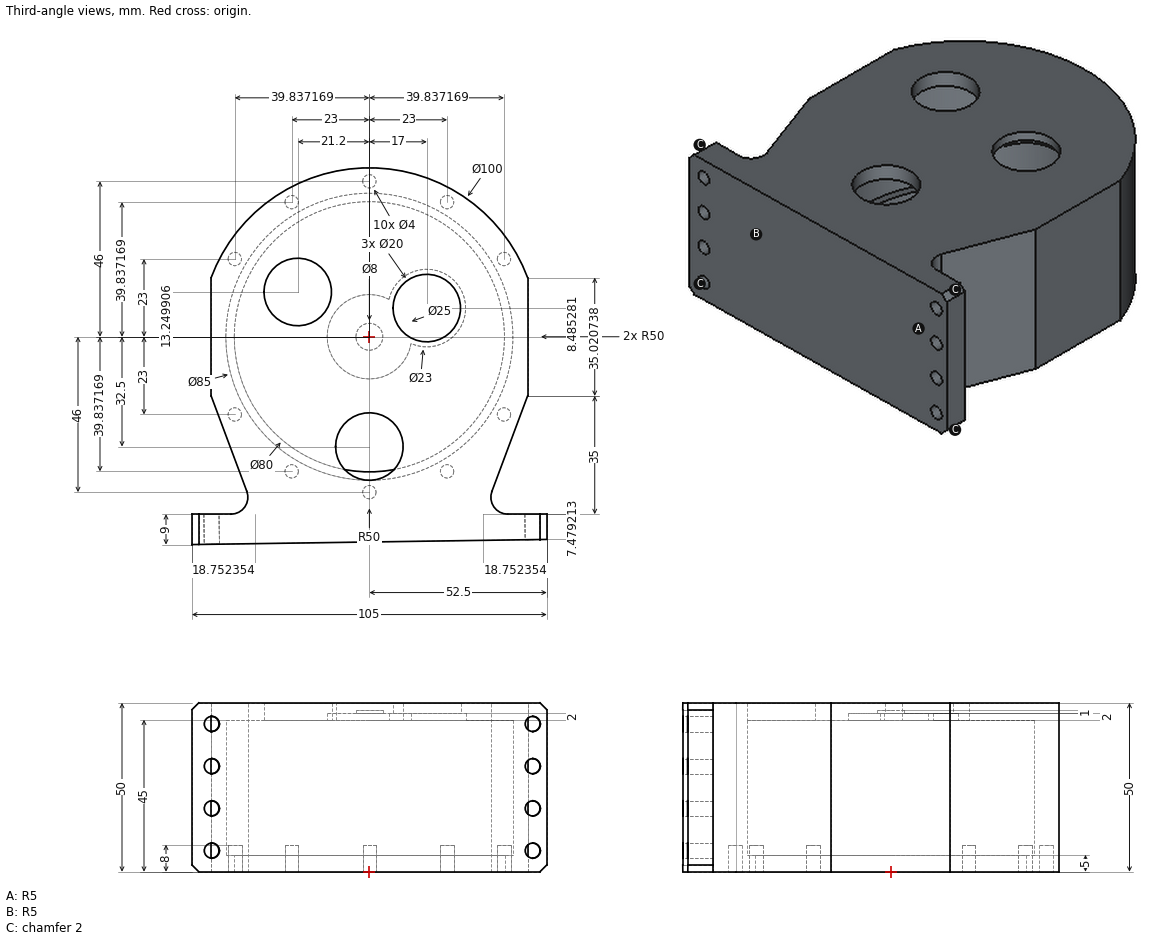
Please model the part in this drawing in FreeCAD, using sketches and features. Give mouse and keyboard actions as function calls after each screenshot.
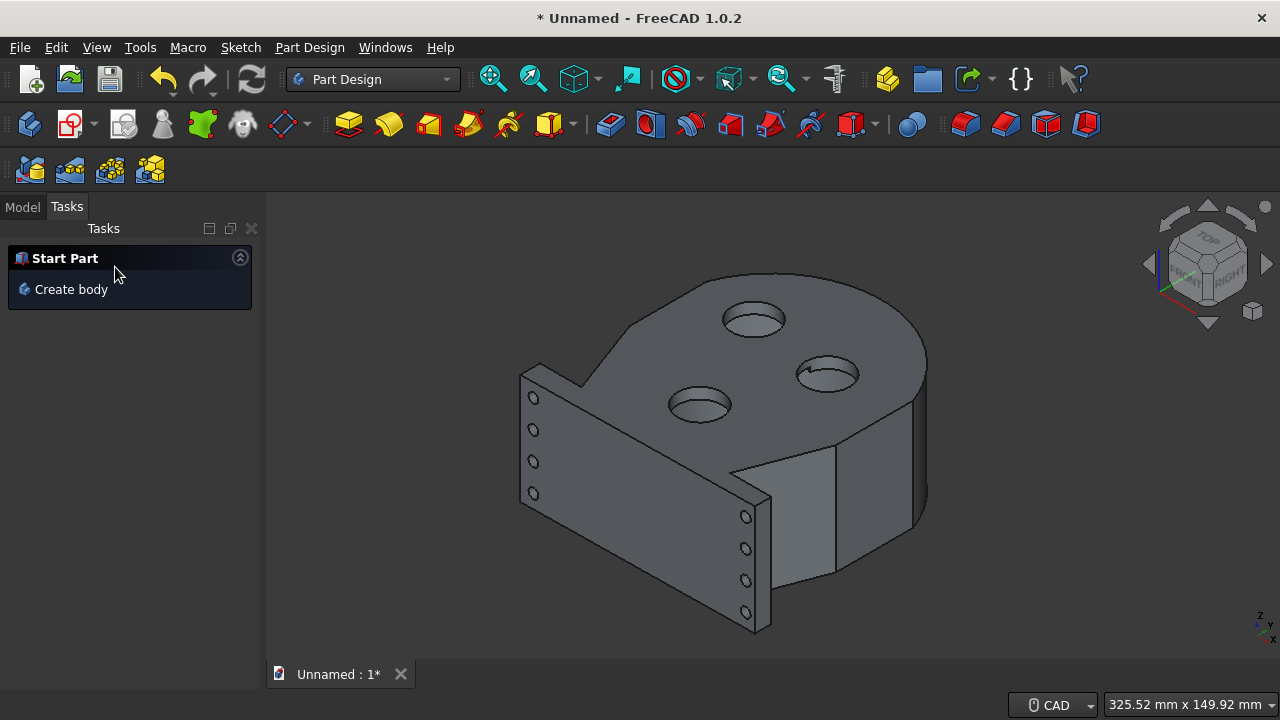
key(1)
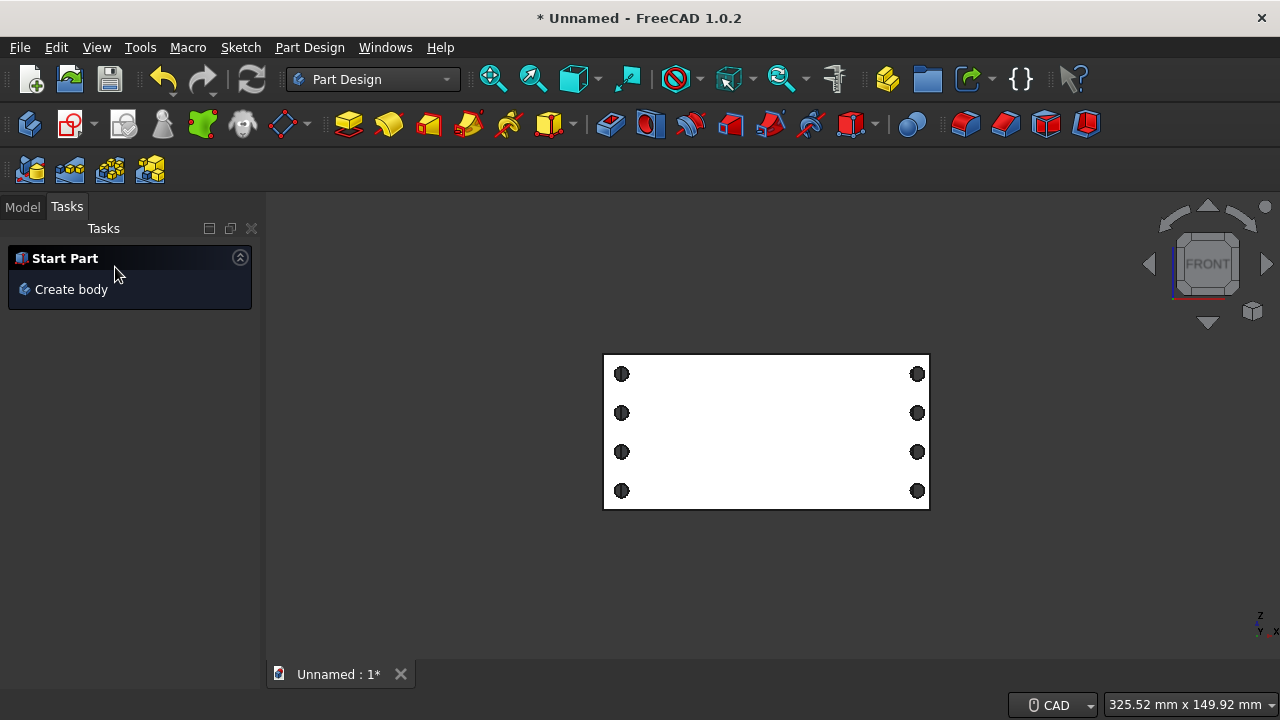
click(494, 80)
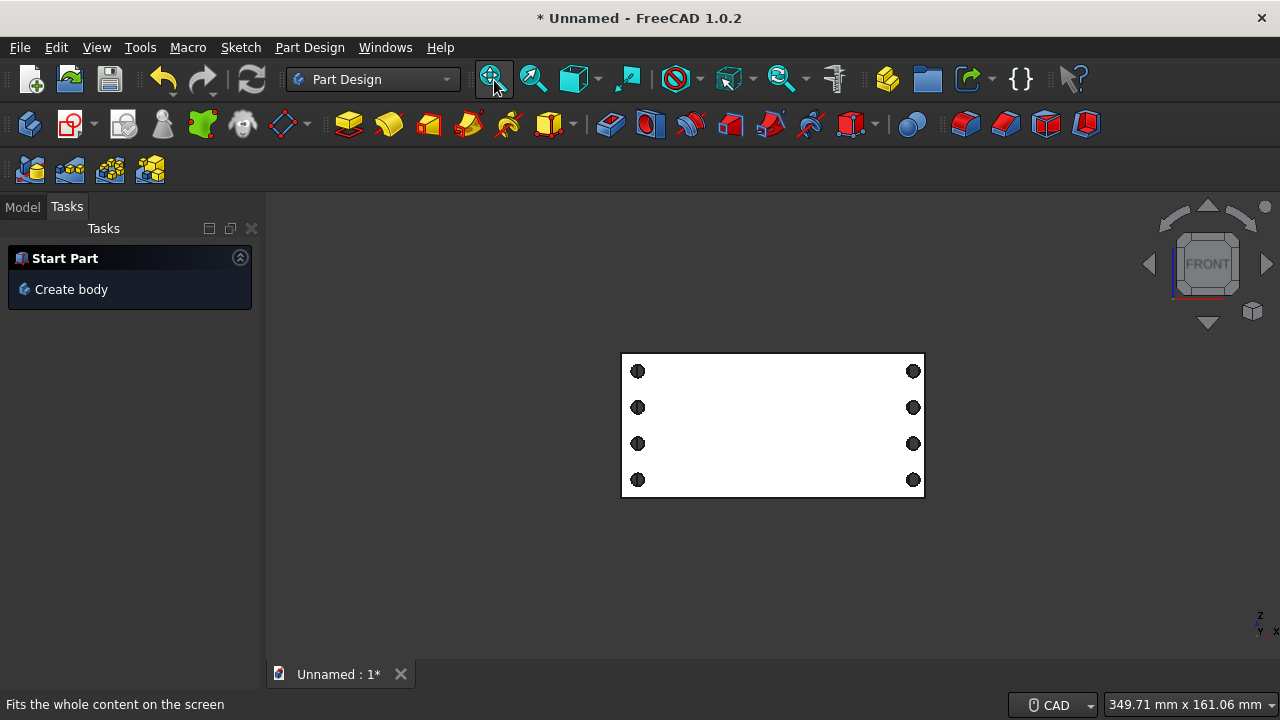
key(3)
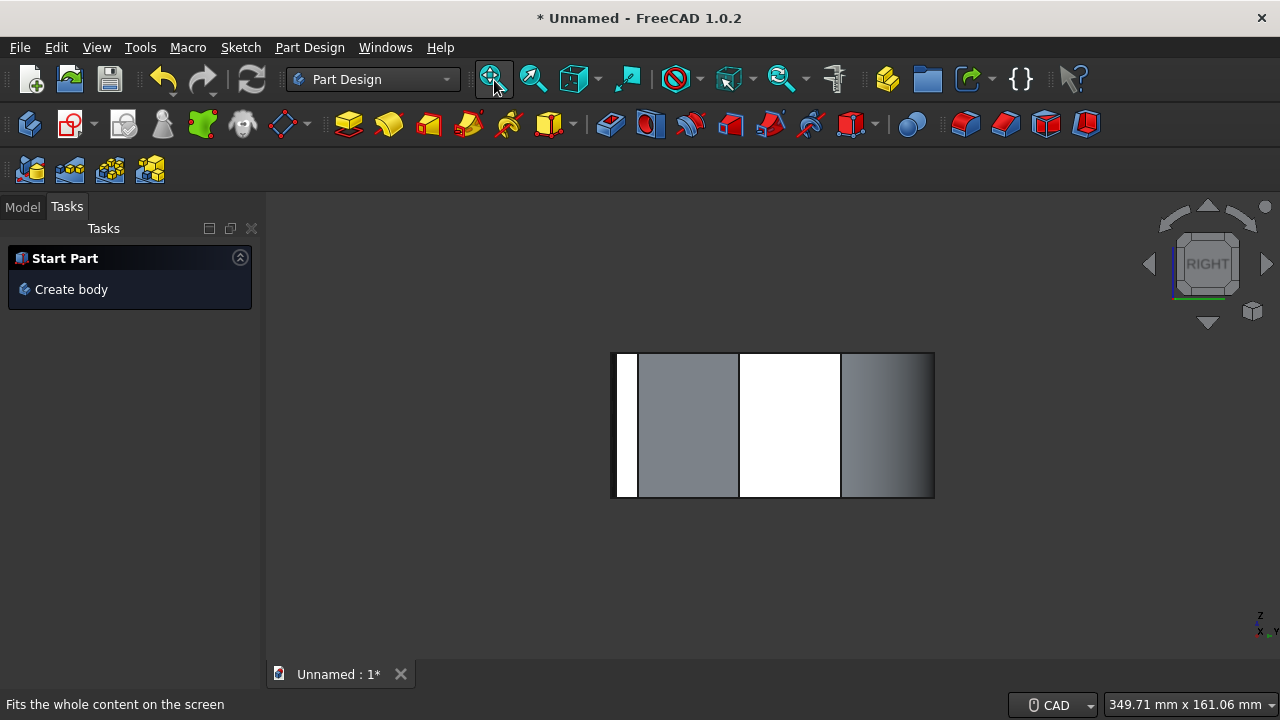
click(494, 80)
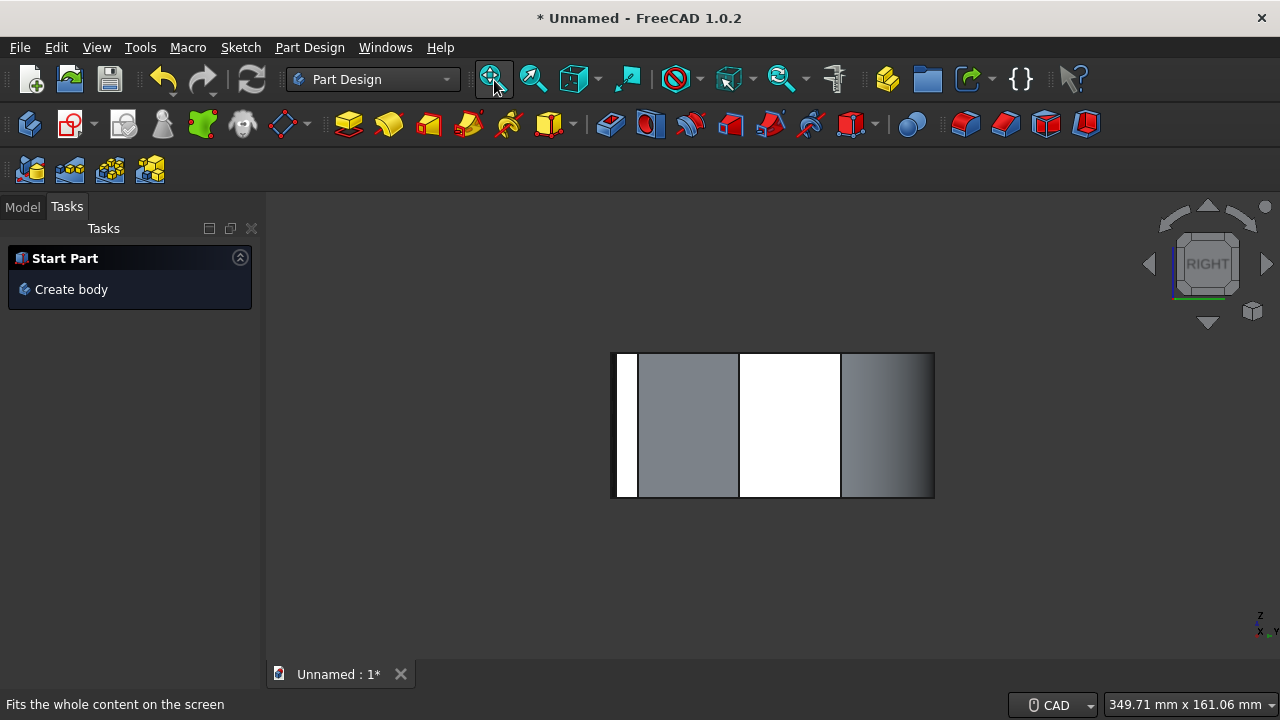
key(5)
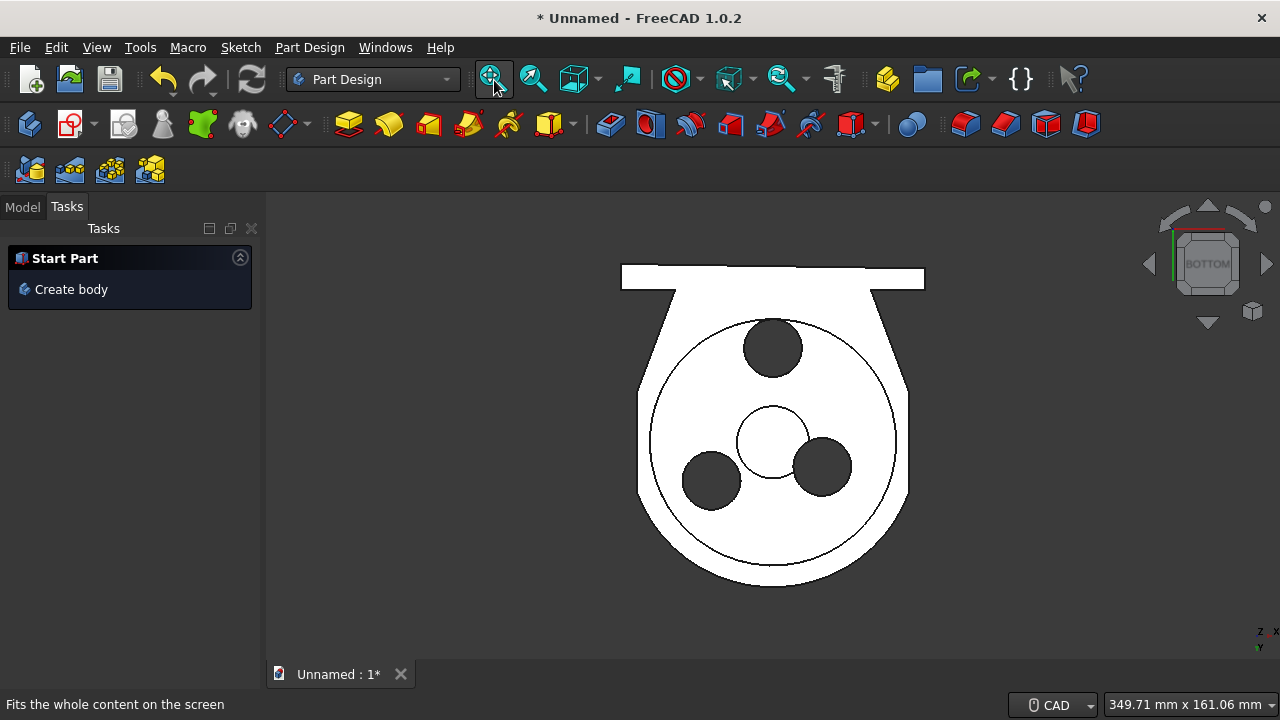
key(4)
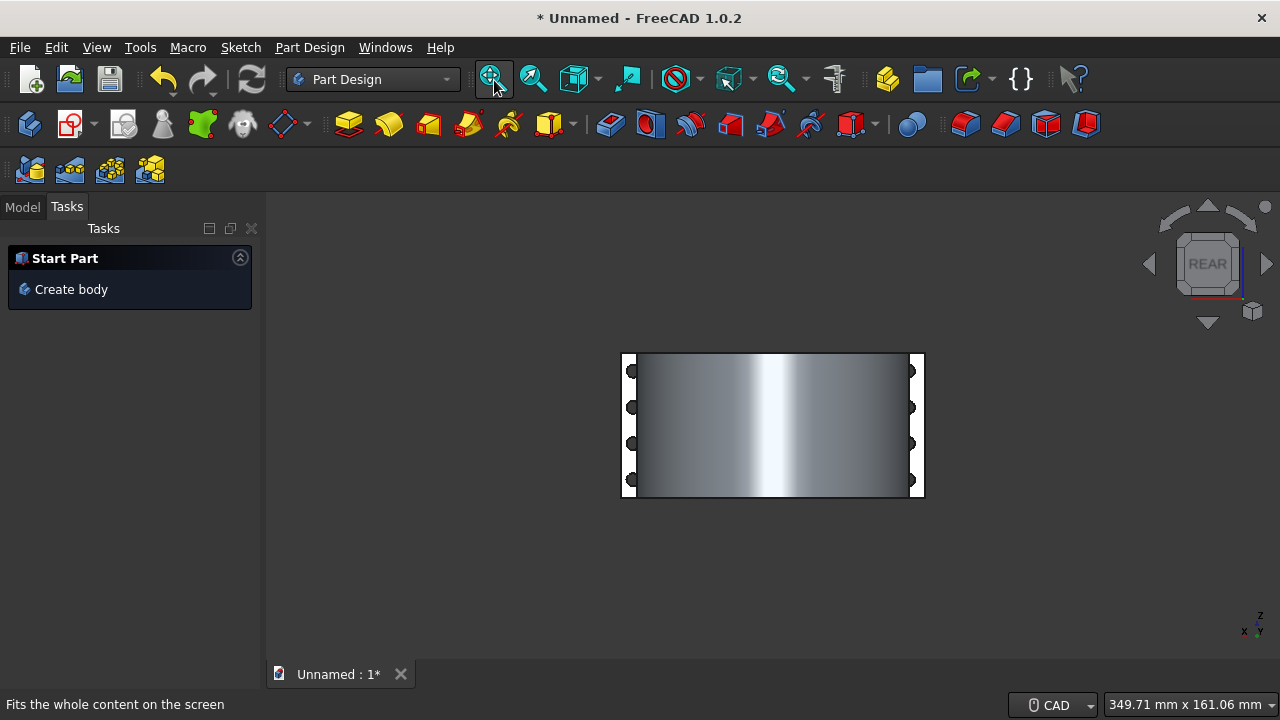
click(494, 80)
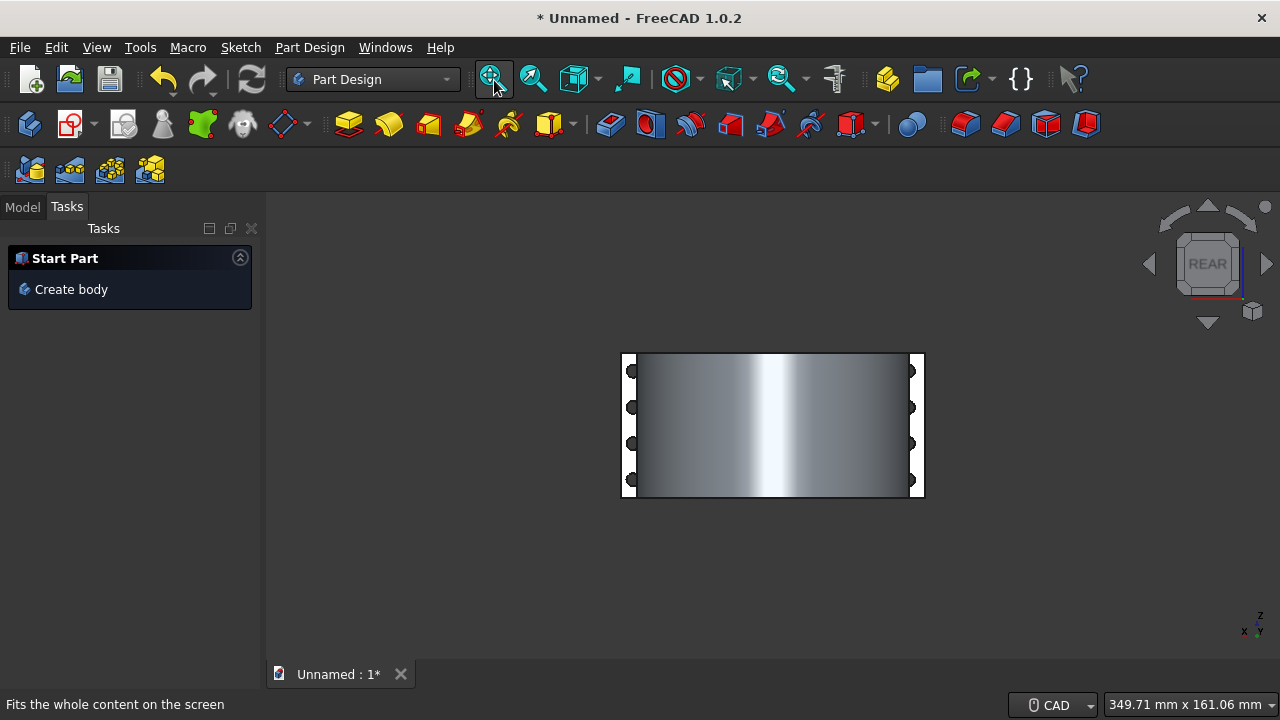
key(6)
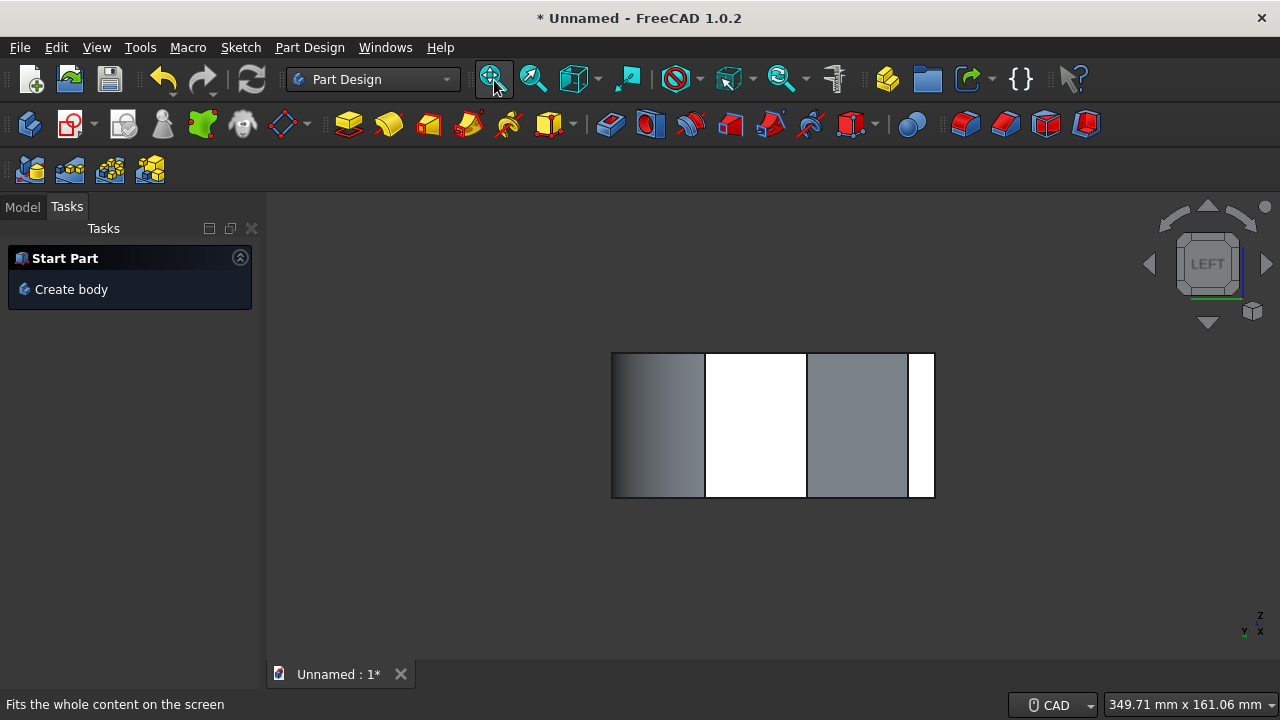
key(v)
key(f)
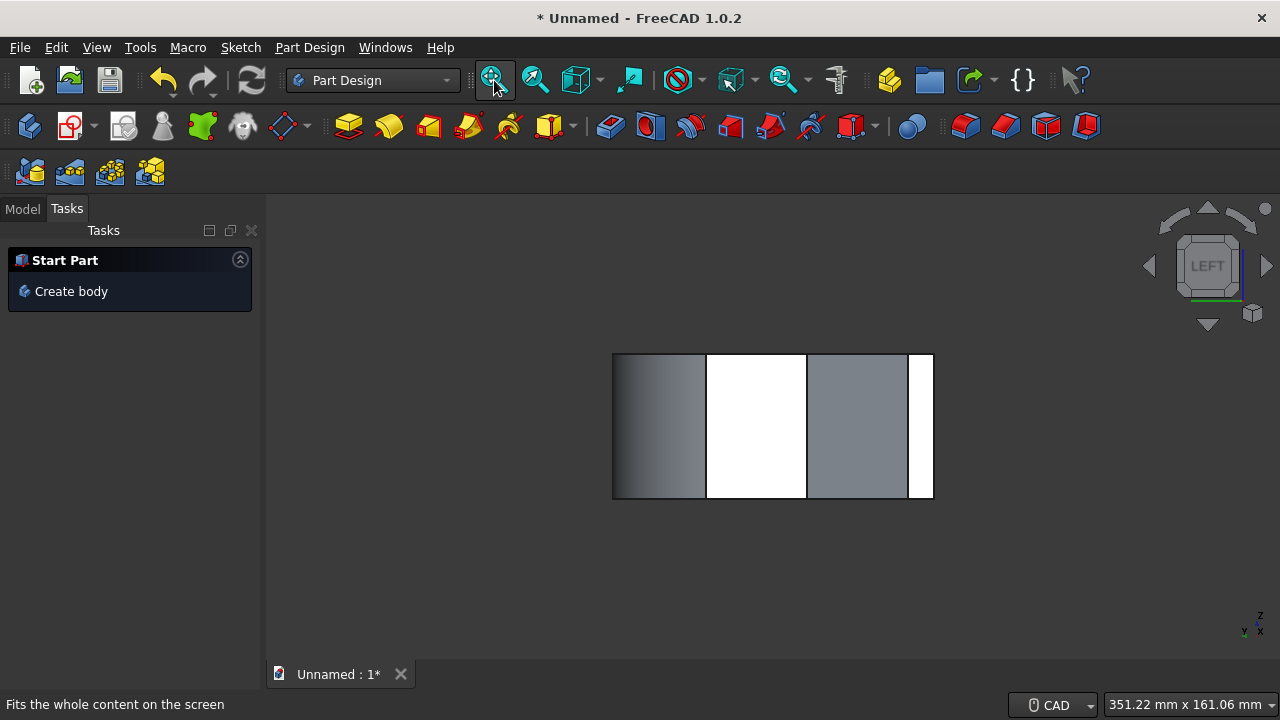
key(v)
key(3)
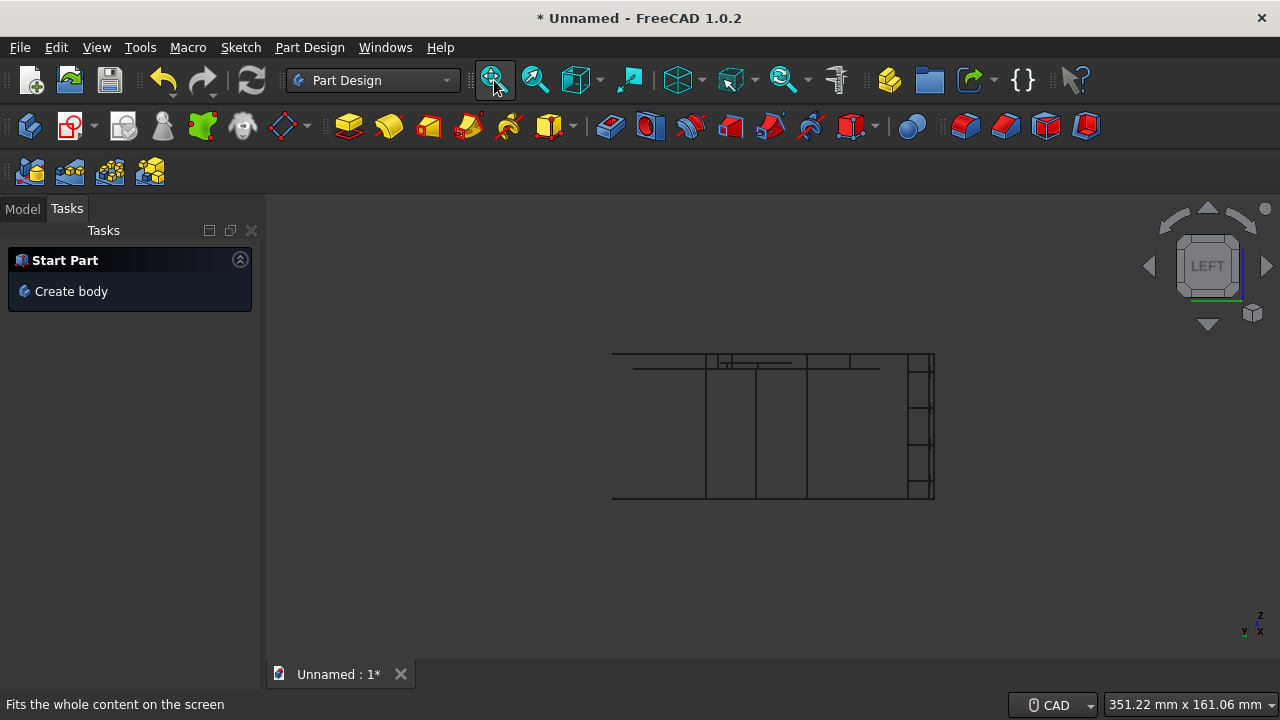
key(0)